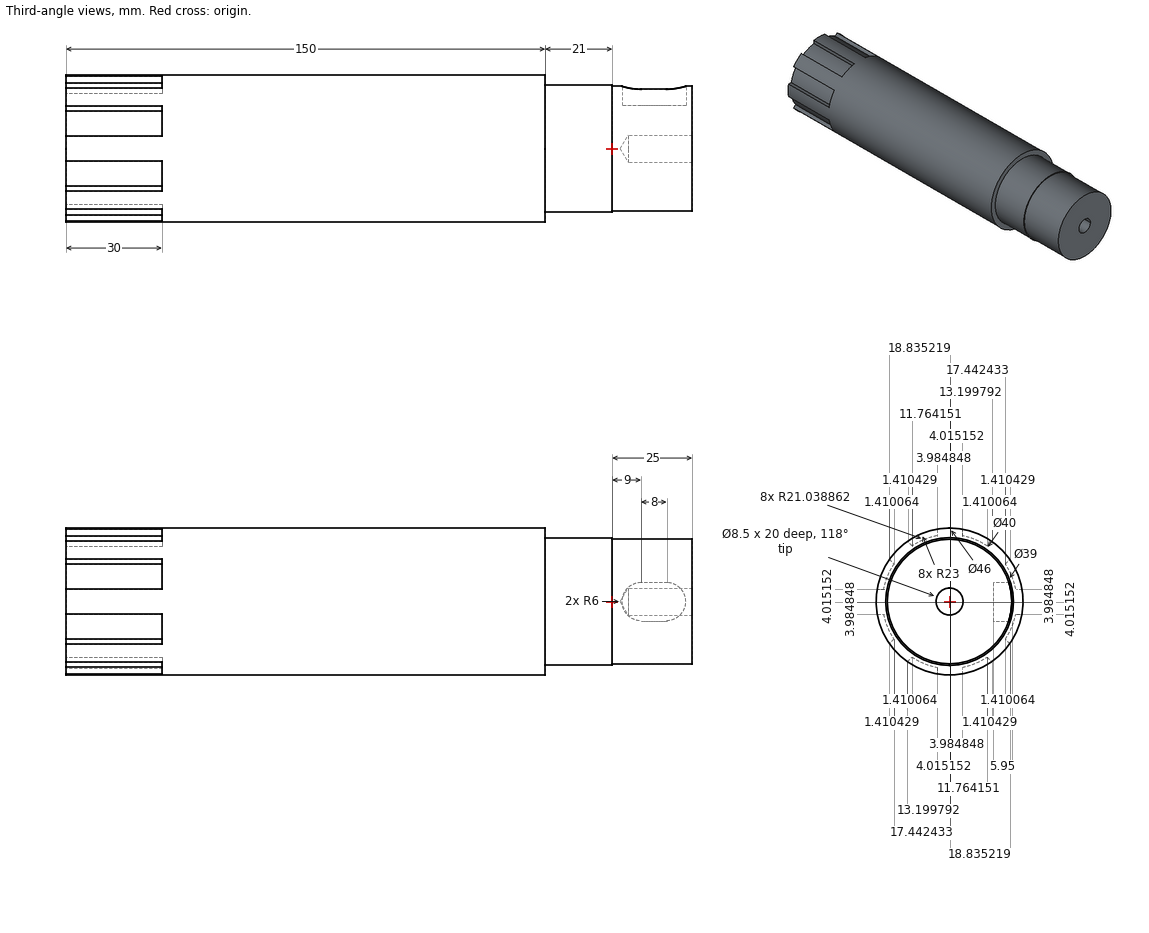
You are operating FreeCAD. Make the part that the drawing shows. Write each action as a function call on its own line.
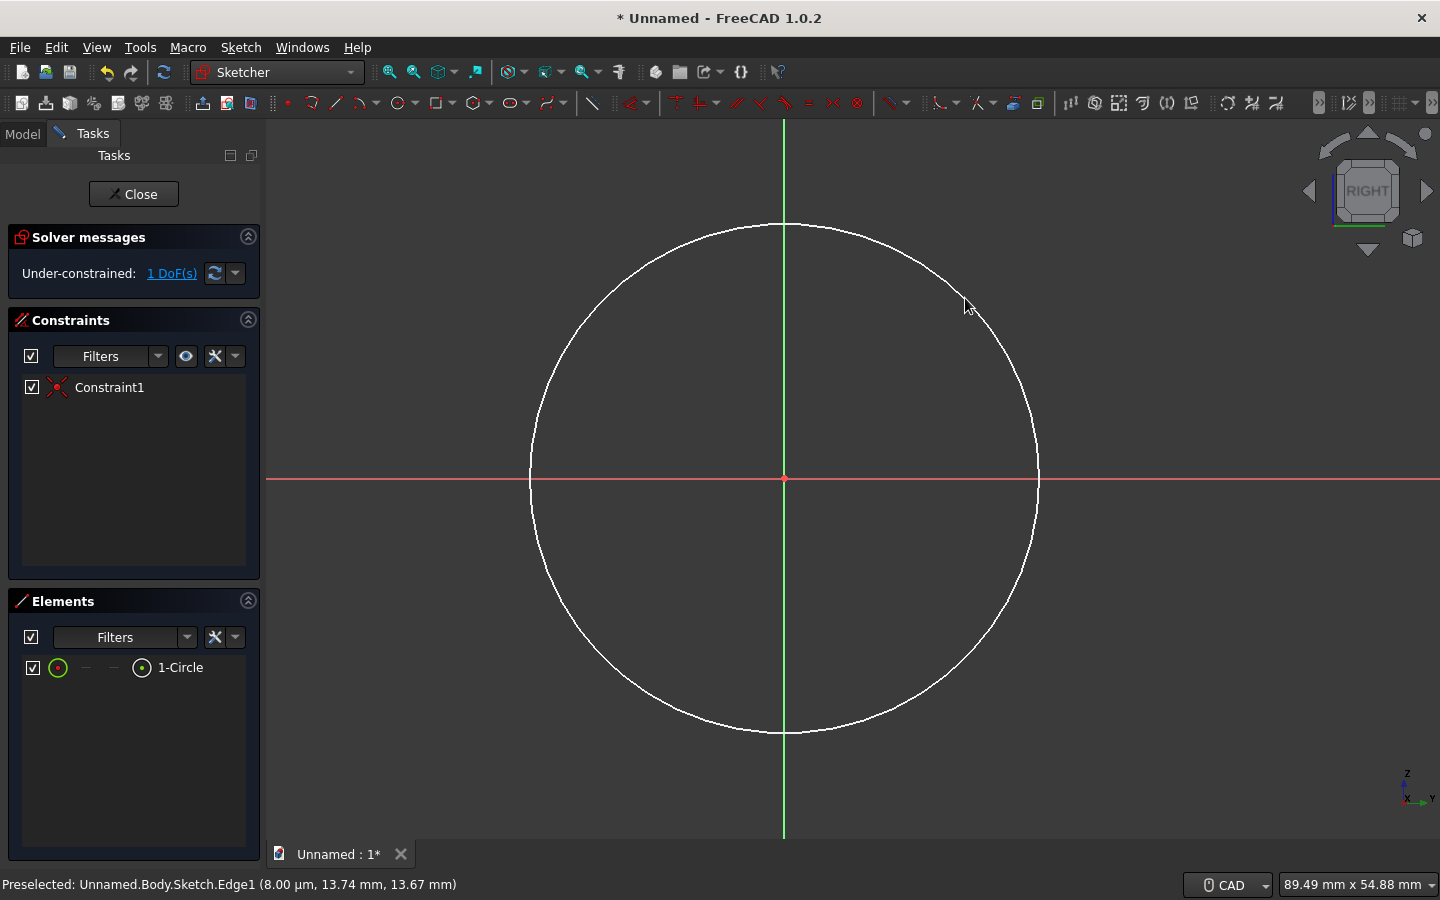
click(630, 104)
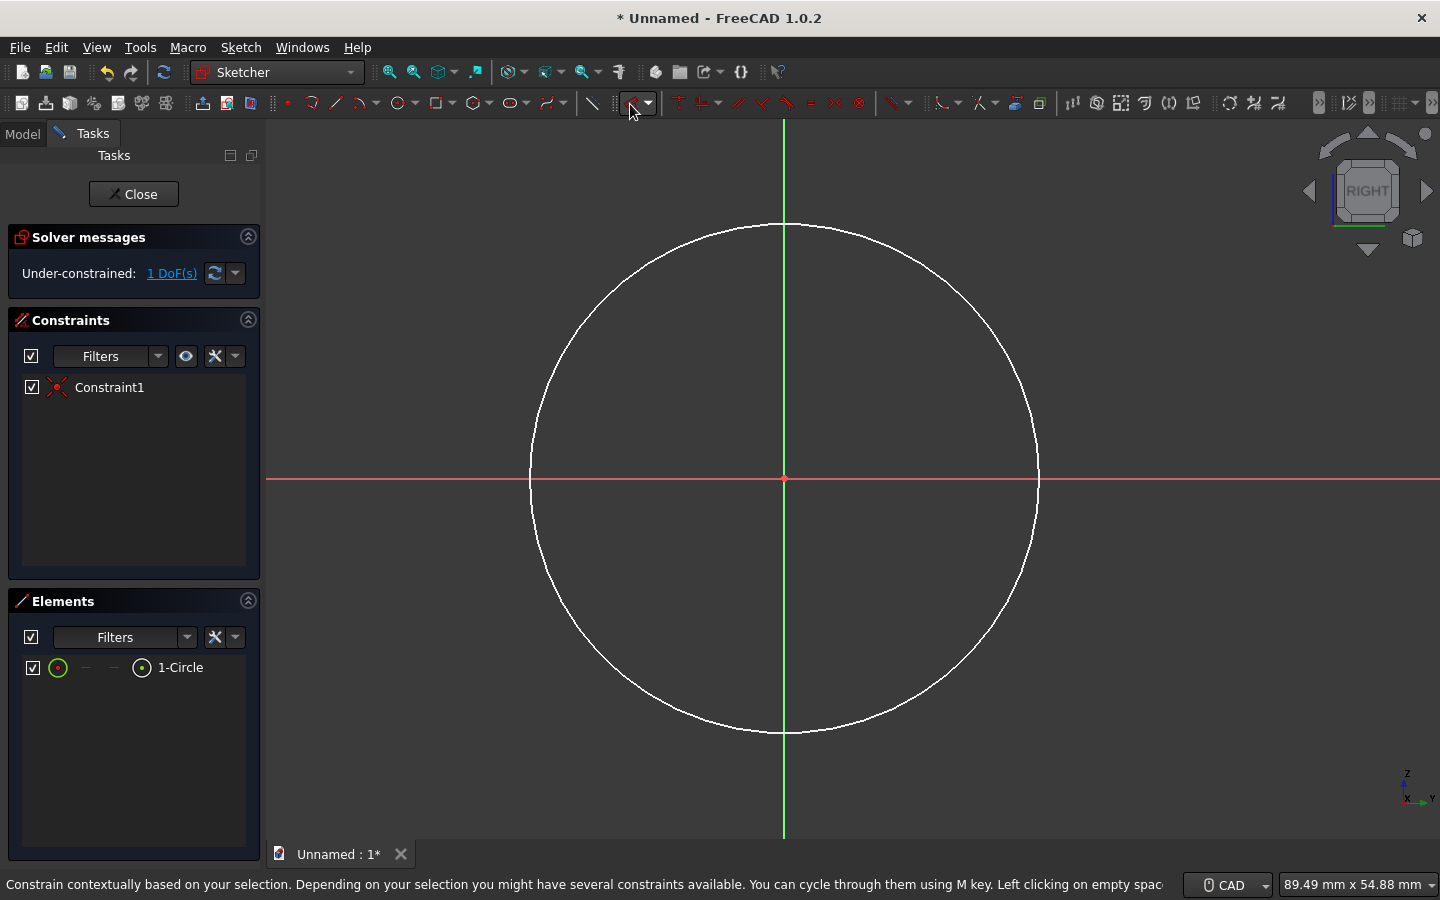
click(964, 298)
click(987, 275)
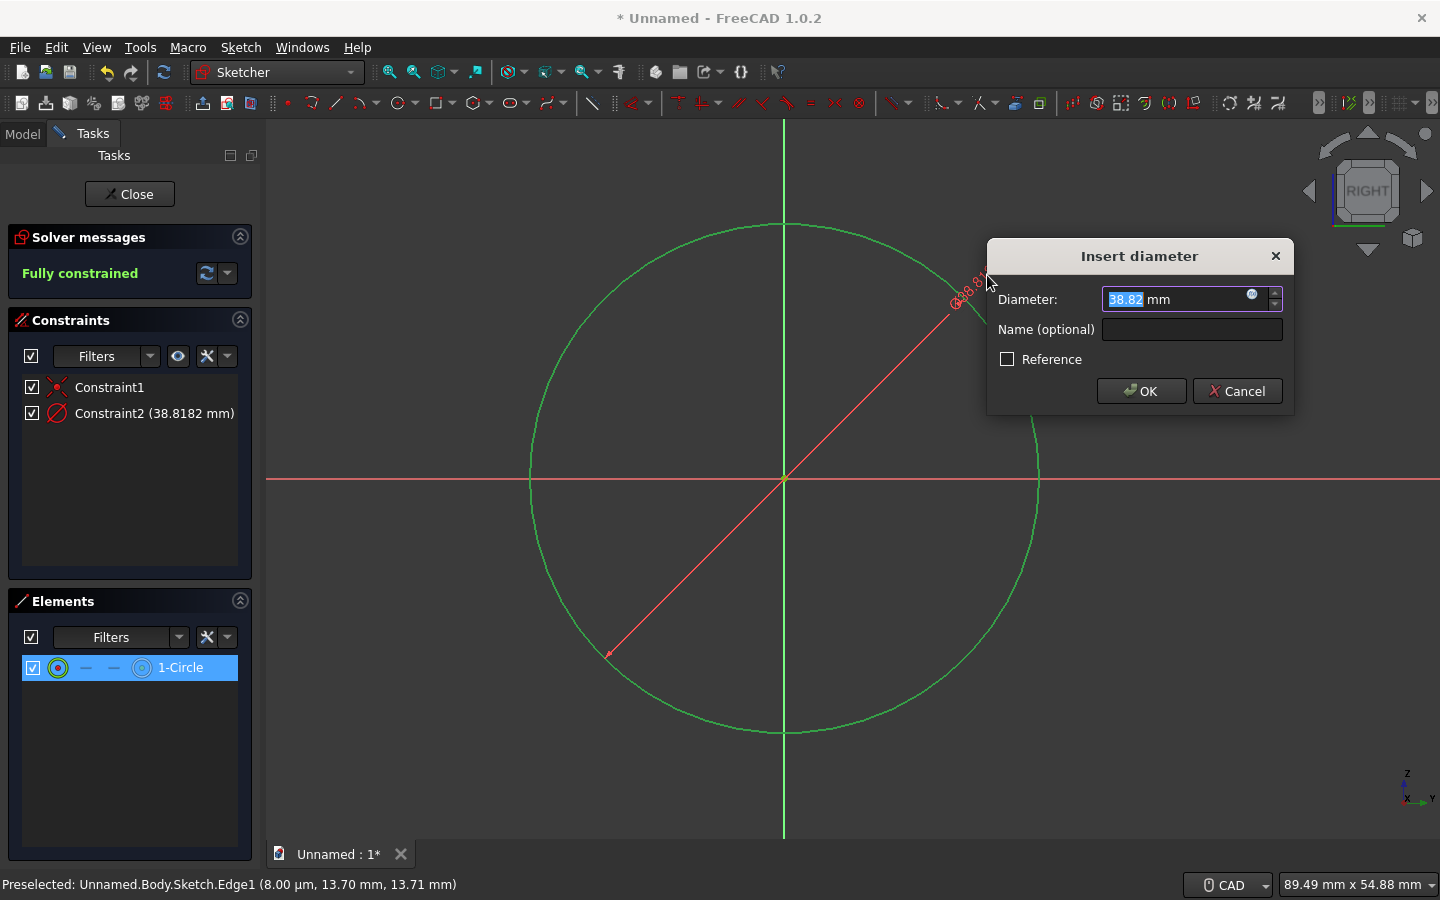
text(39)
key(Return)
key(Escape)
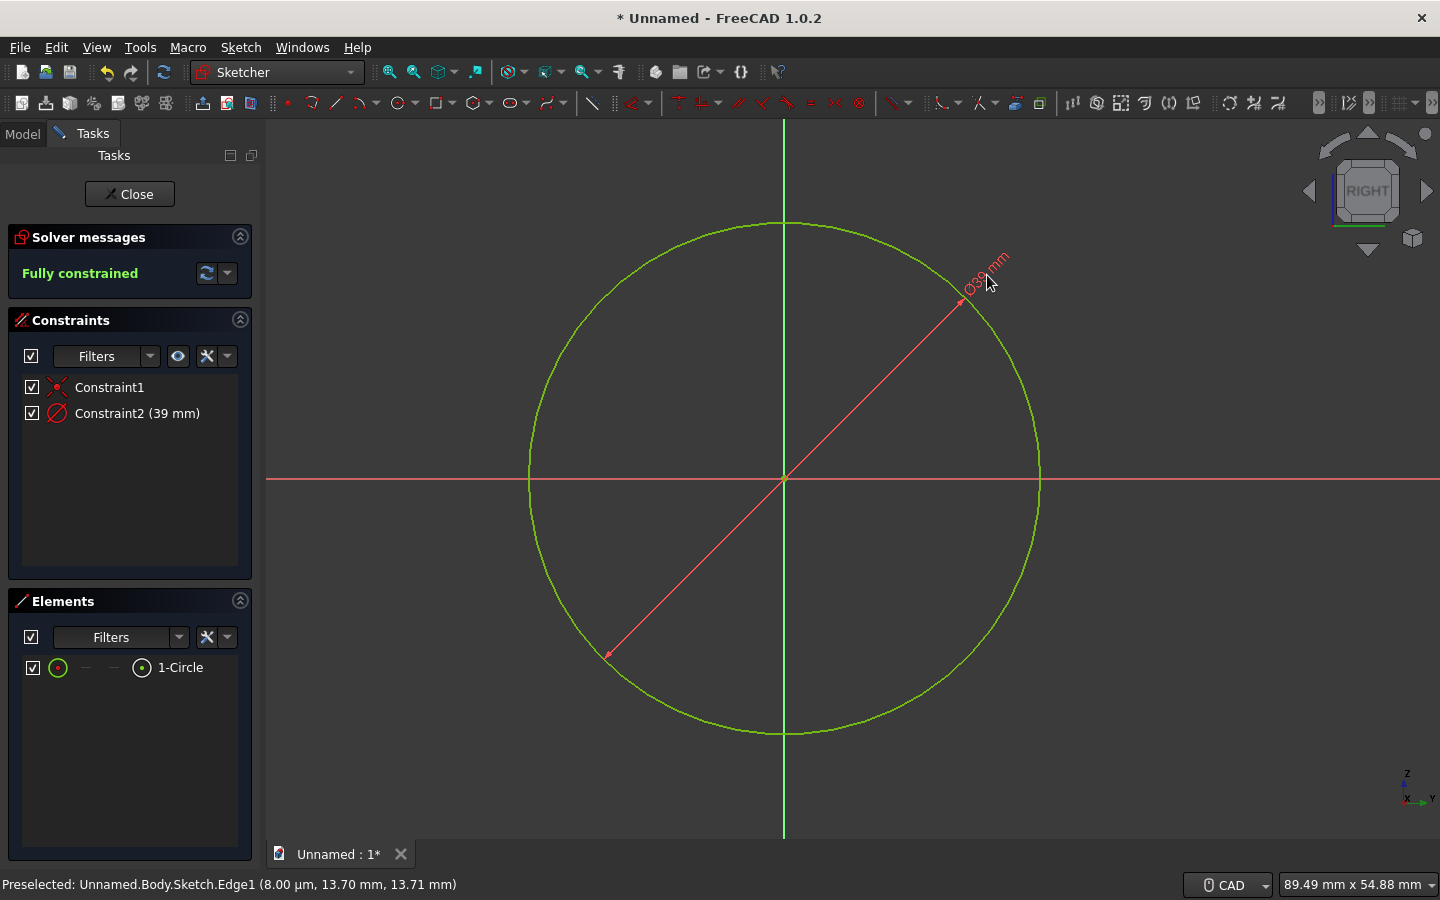
click(130, 194)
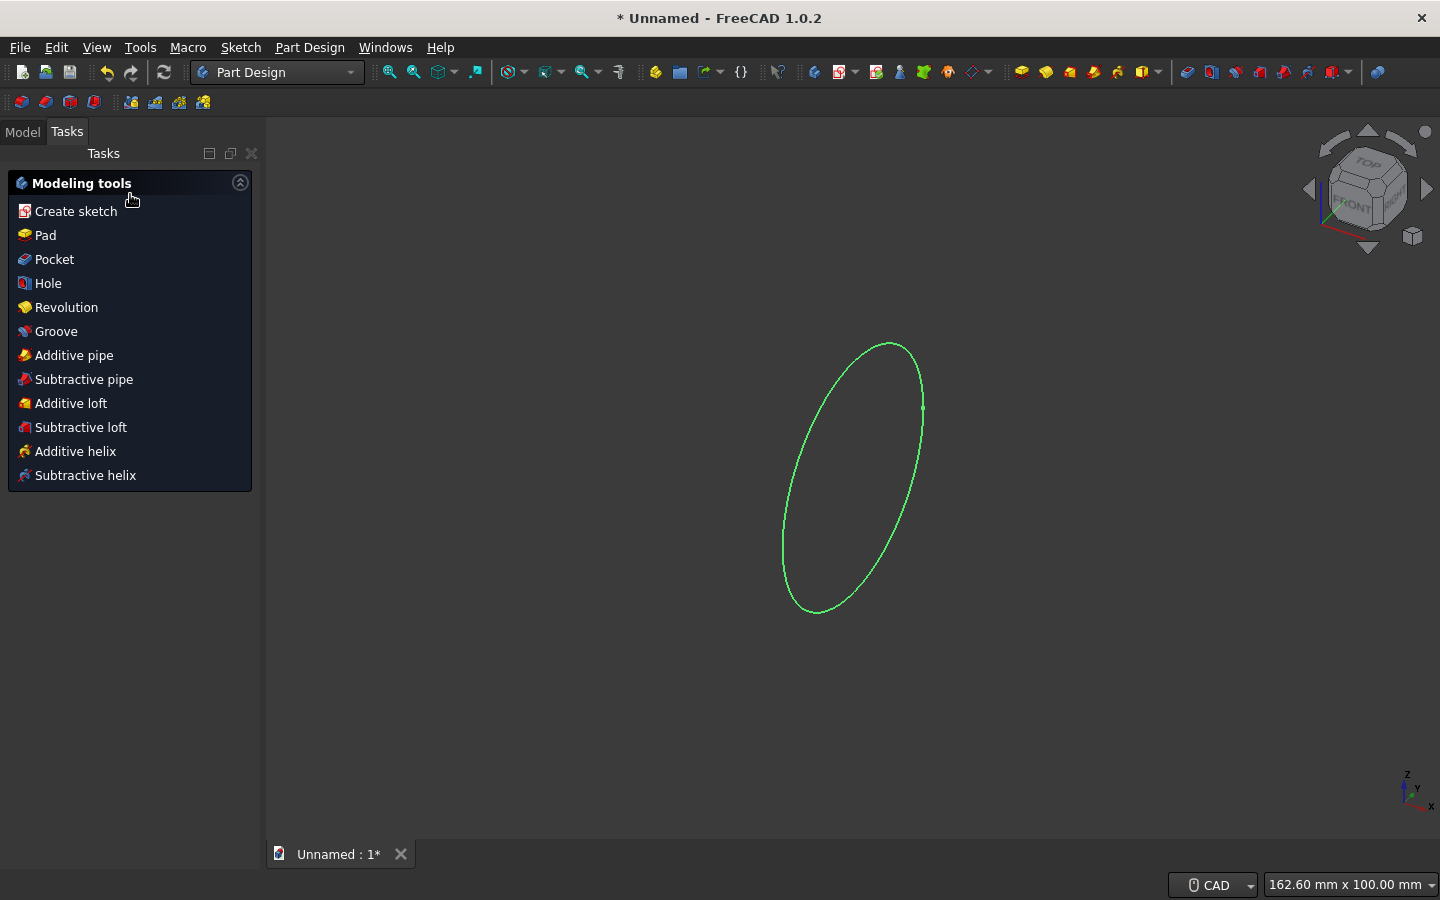
click(1022, 72)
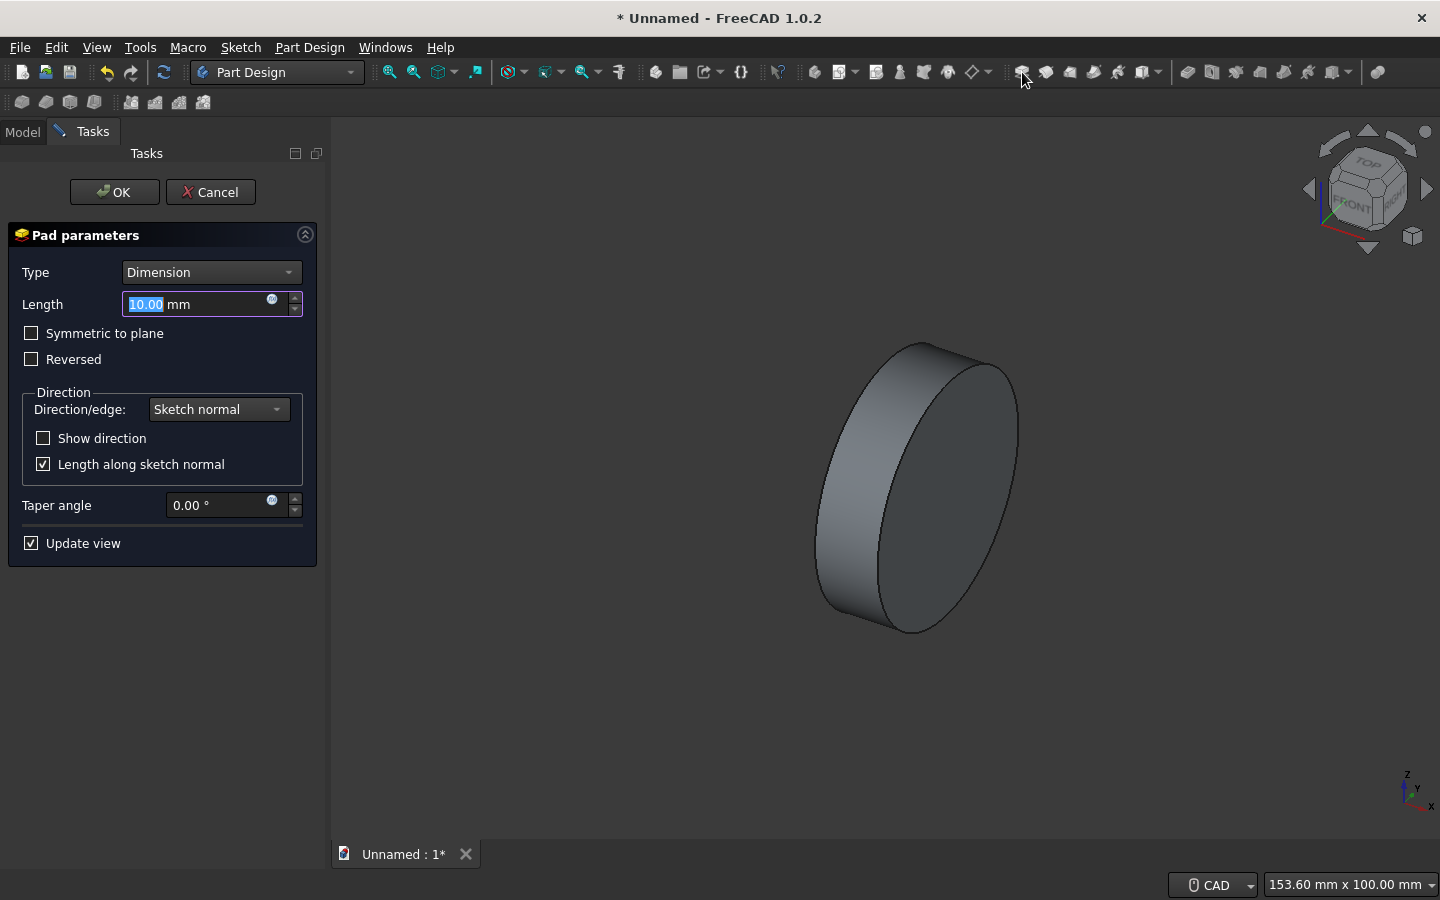
text(25)
key(Tab)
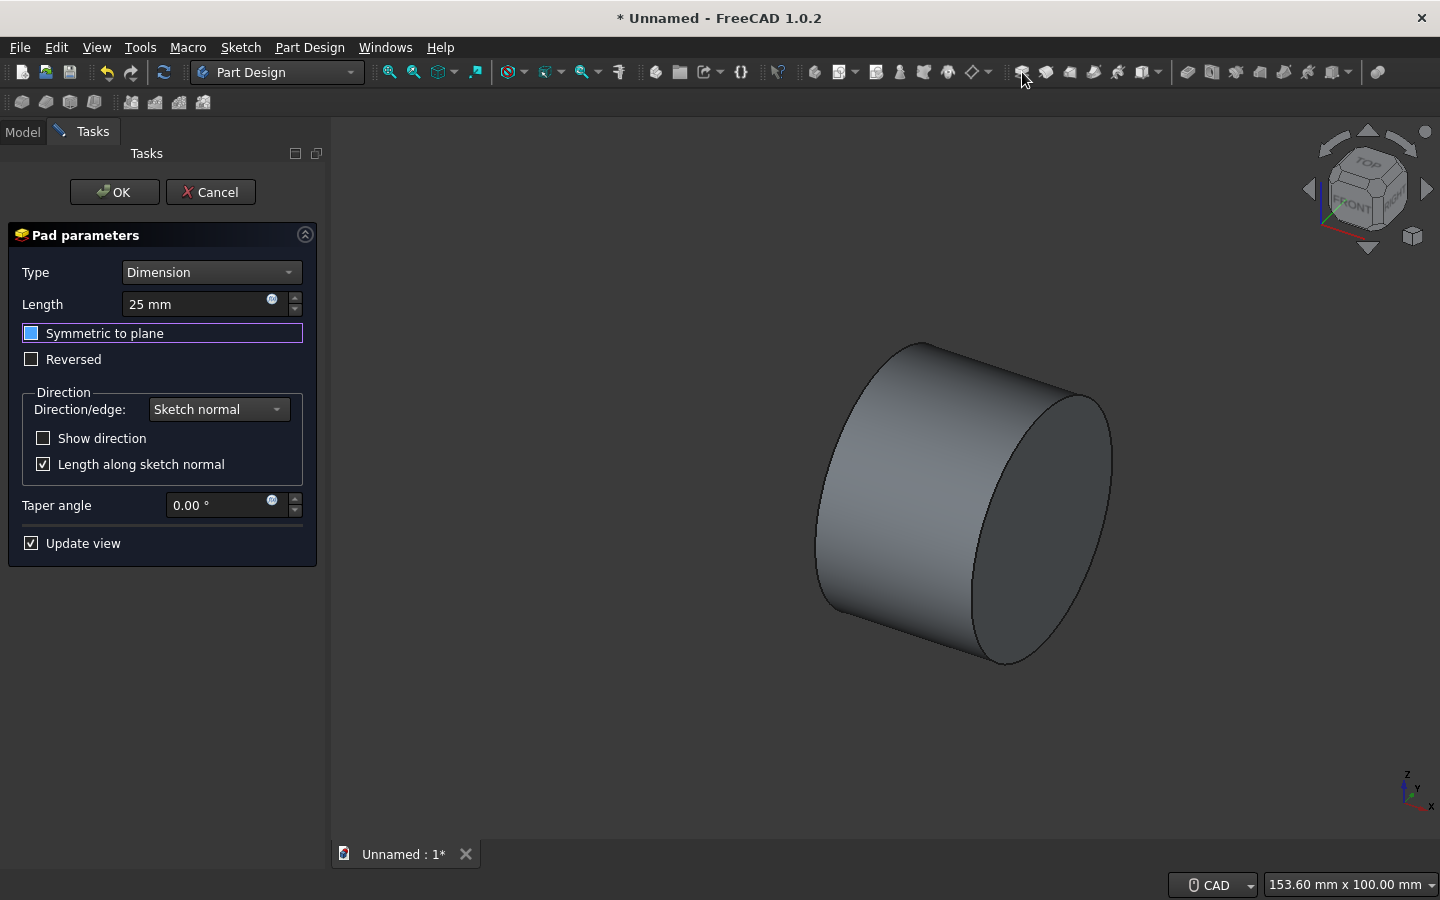
click(115, 192)